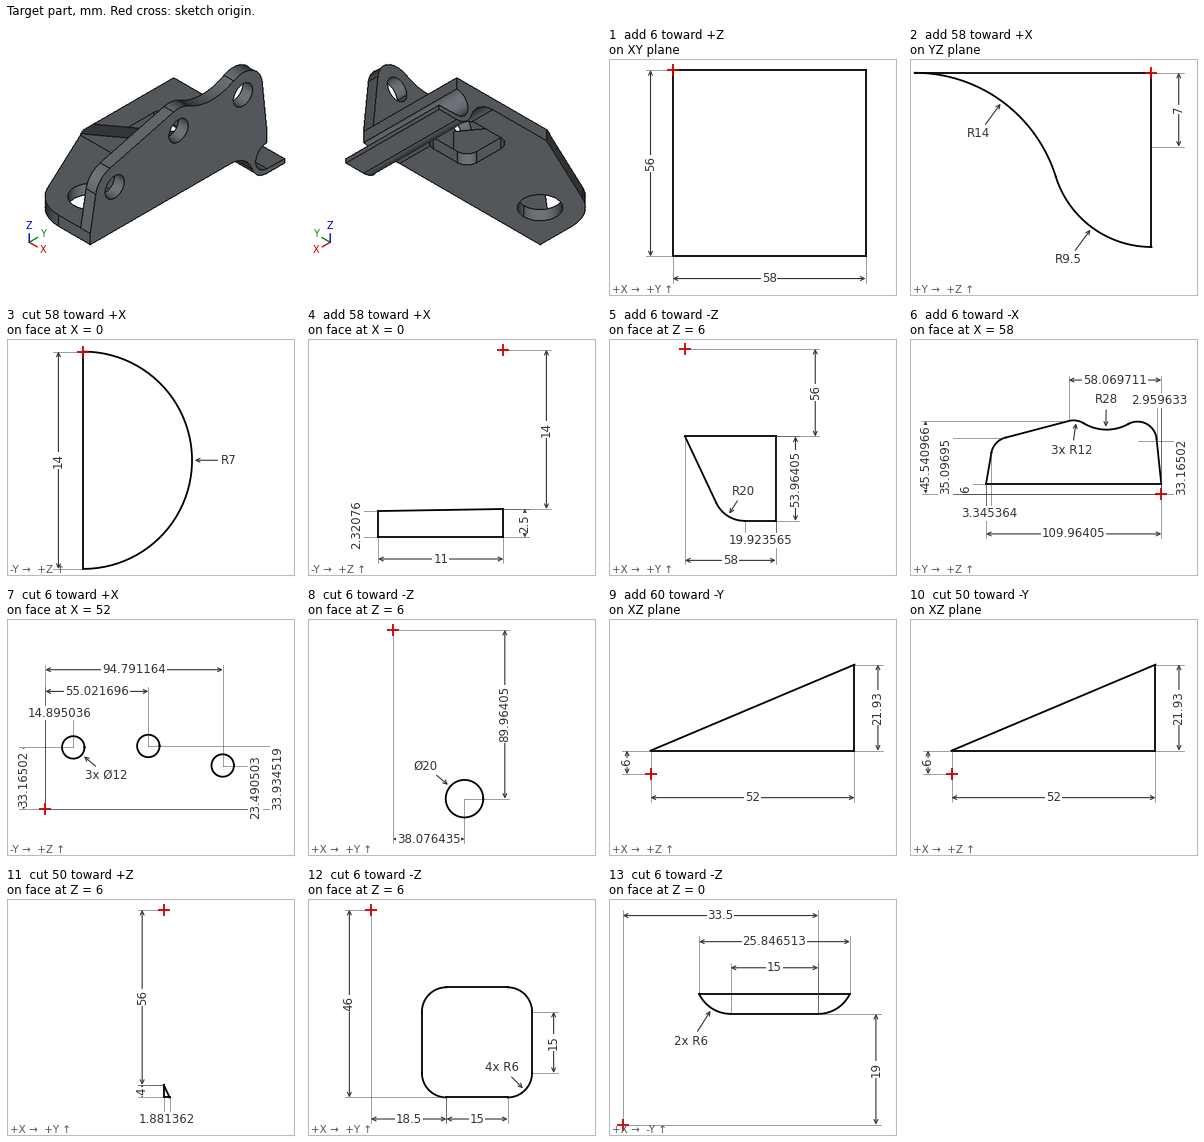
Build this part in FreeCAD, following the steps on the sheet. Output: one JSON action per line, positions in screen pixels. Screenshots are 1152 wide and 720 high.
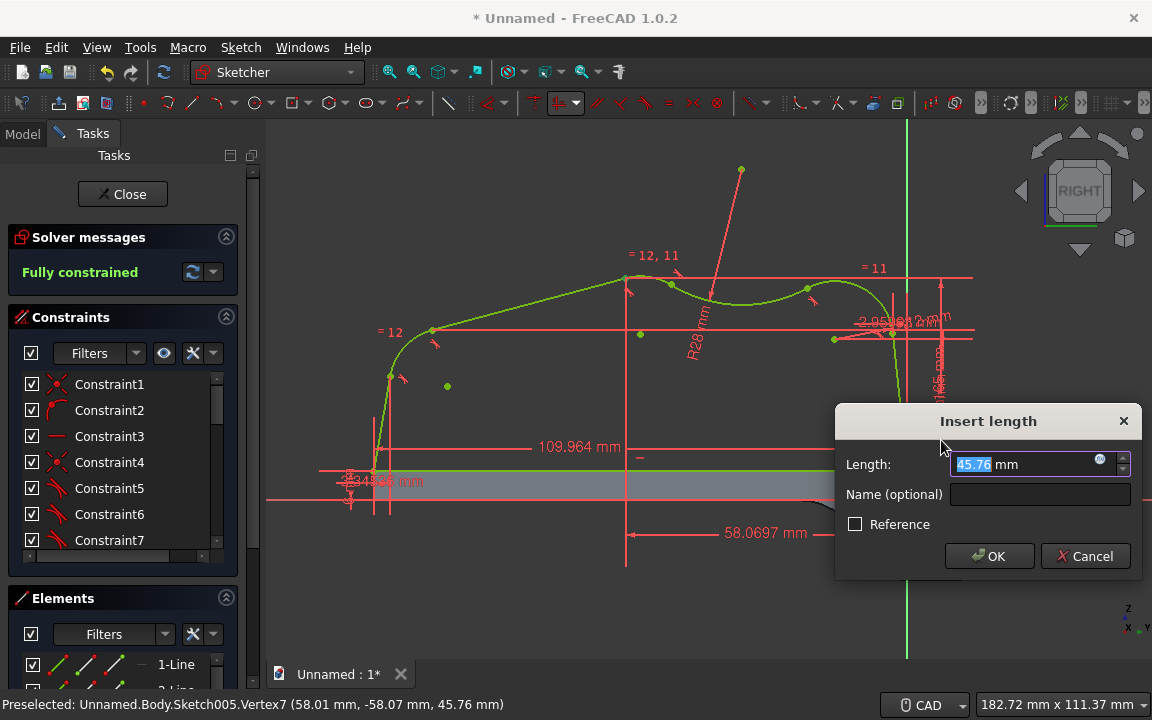
{"action": "type", "text": "45.540966"}
{"action": "key", "text": "Return"}
{"action": "key", "text": "Escape"}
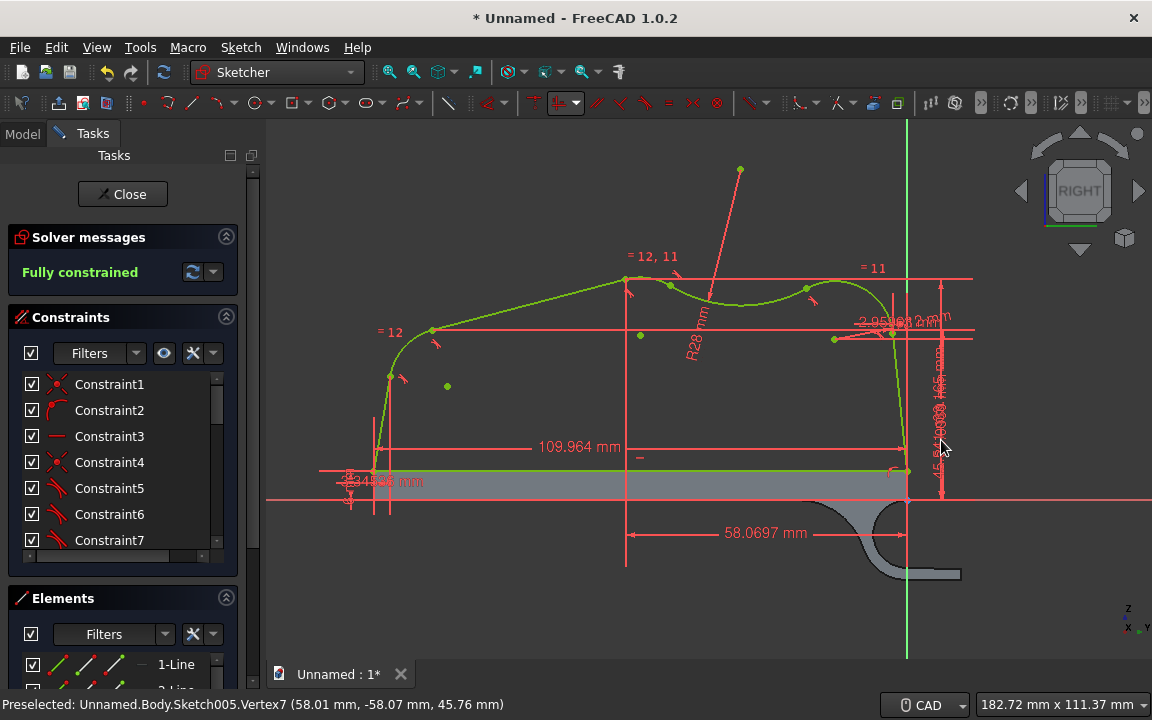
{"action": "left_click", "coordinate": [123, 194]}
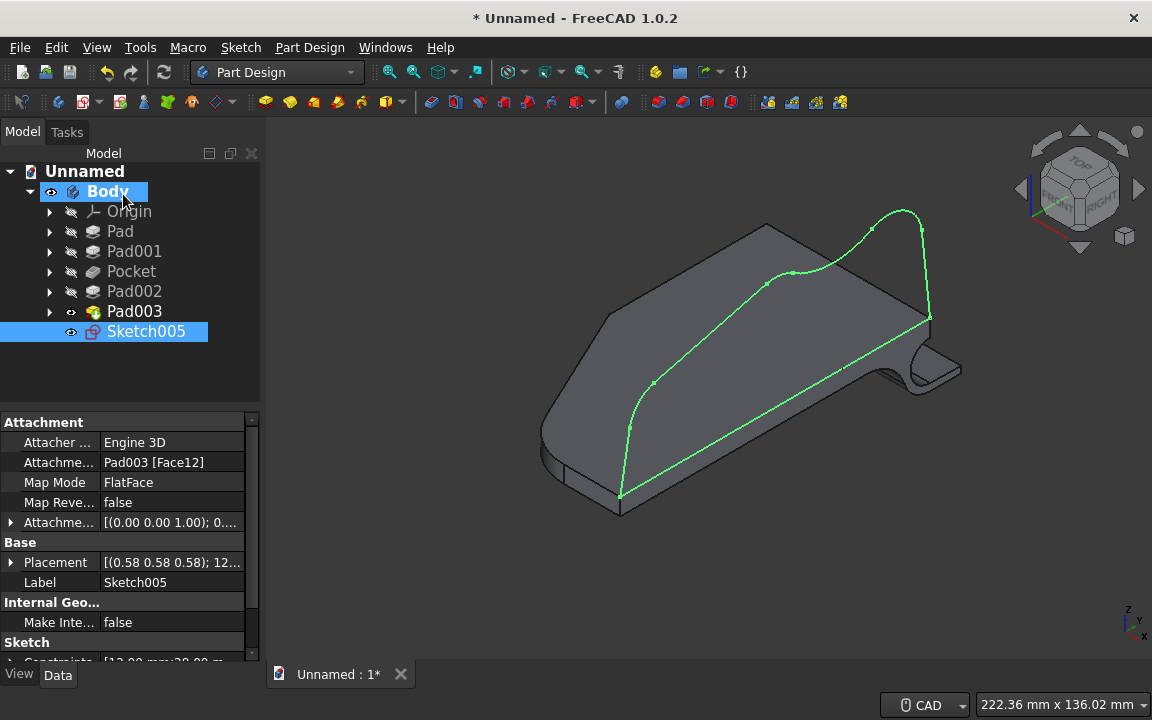
{"action": "left_click", "coordinate": [266, 102]}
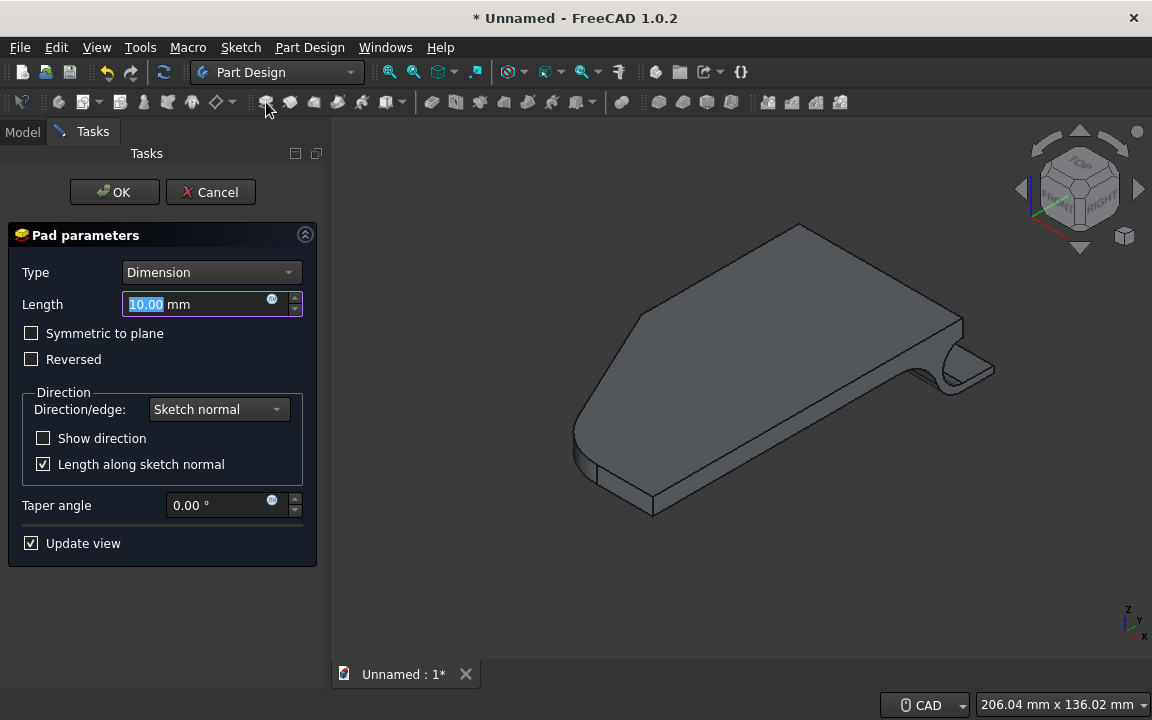
{"action": "type", "text": "6"}
{"action": "key", "text": "Tab"}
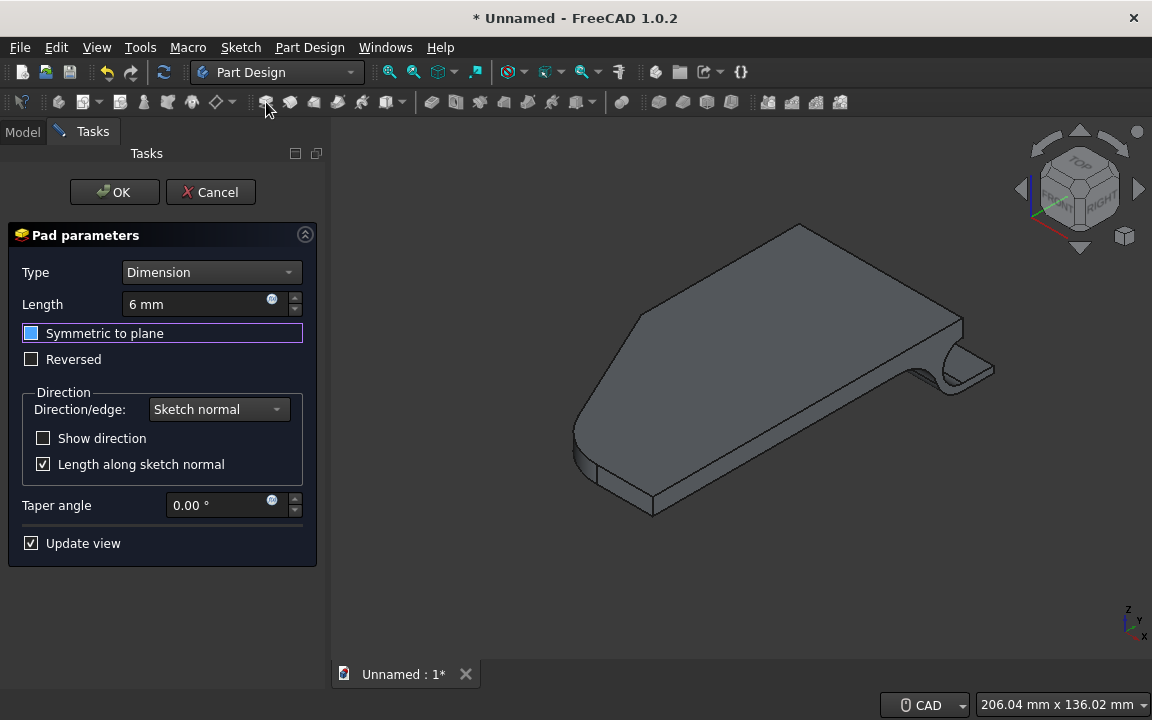
{"action": "left_click", "coordinate": [30, 359]}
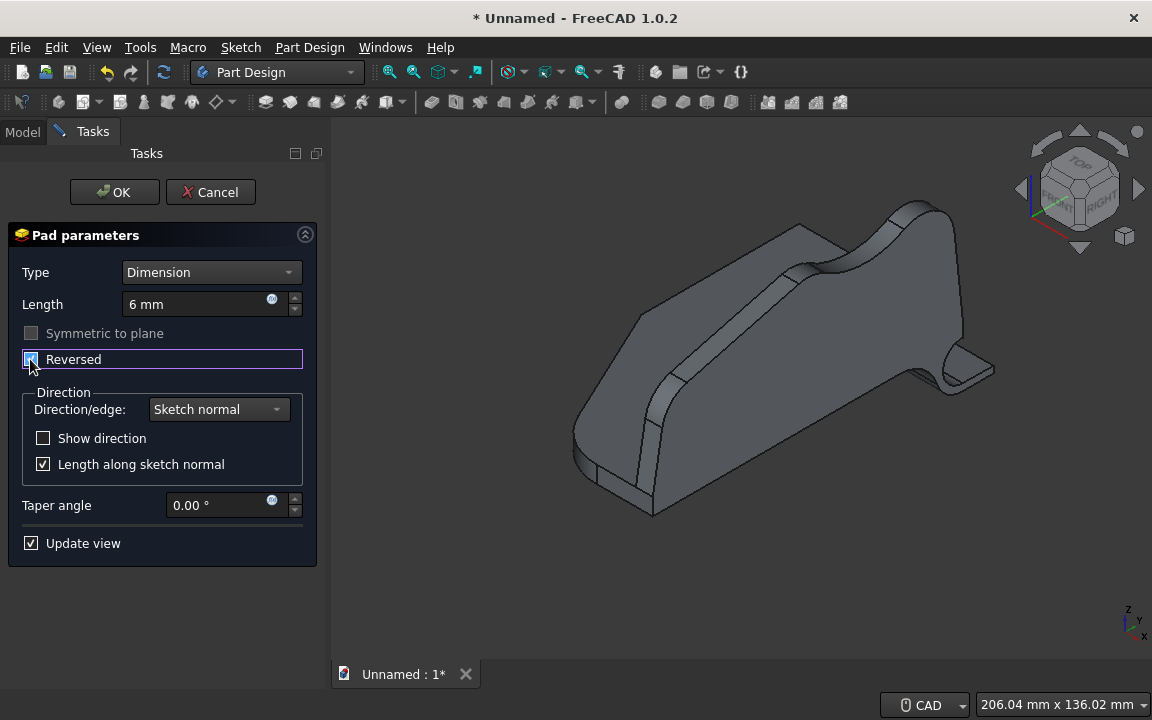
{"action": "left_click", "coordinate": [115, 192]}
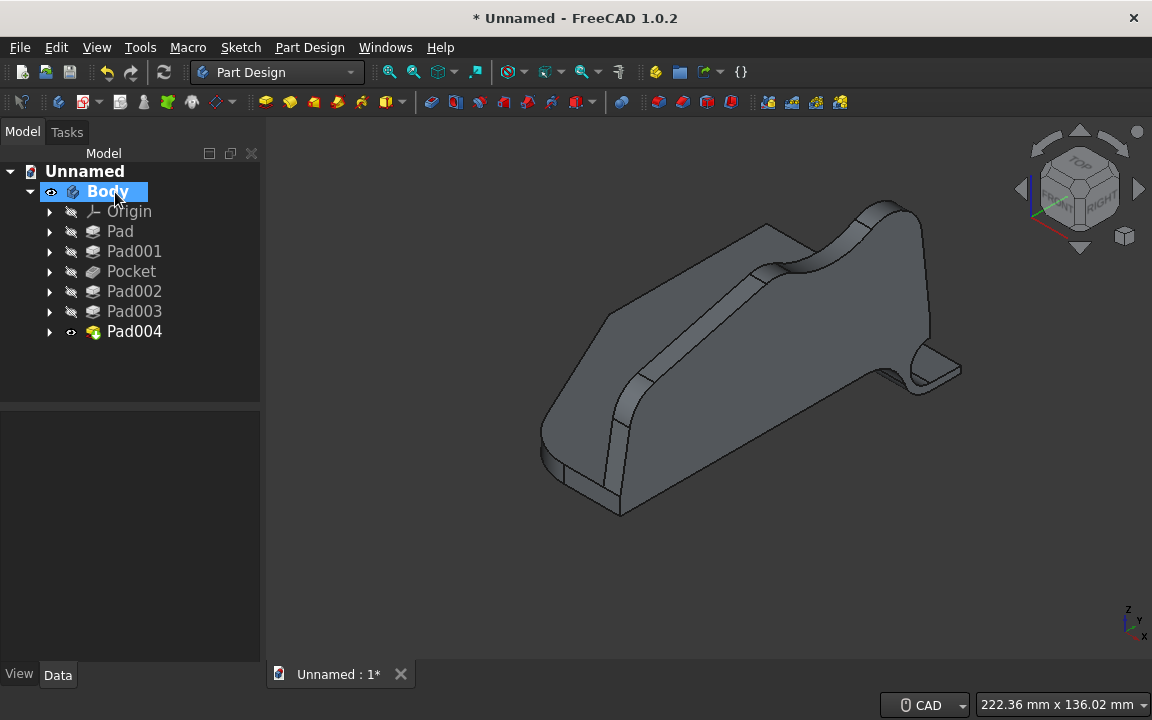
{"action": "left_click", "coordinate": [390, 72]}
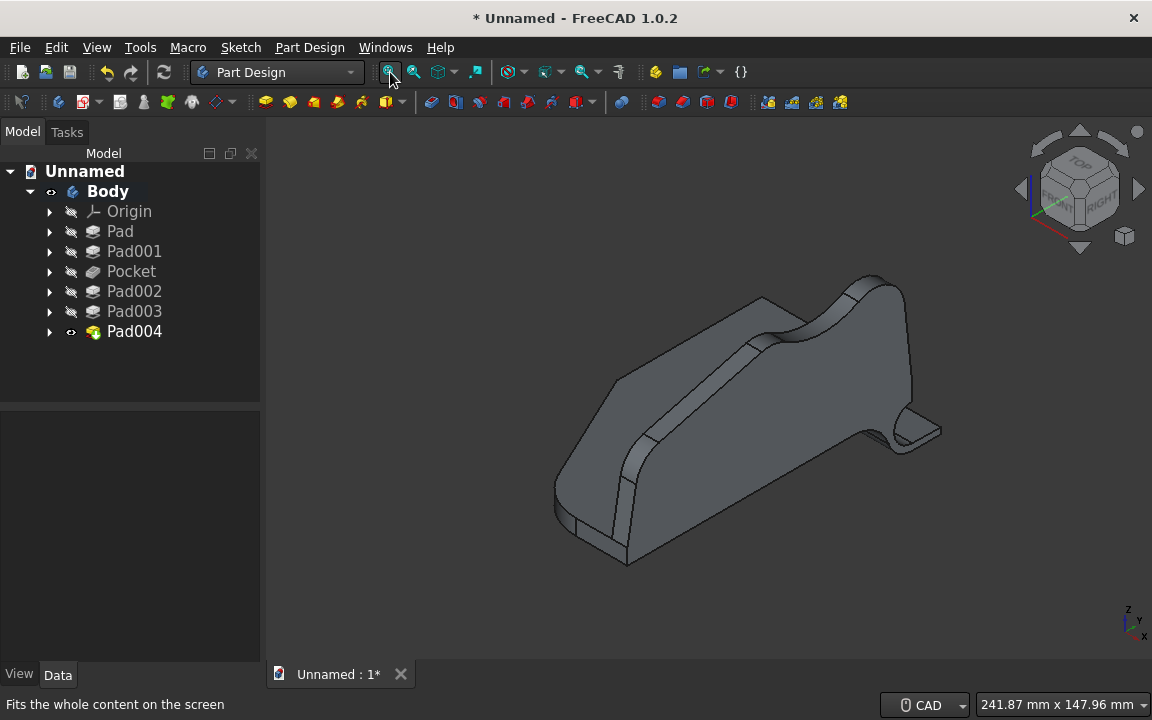
{"action": "key", "text": "6"}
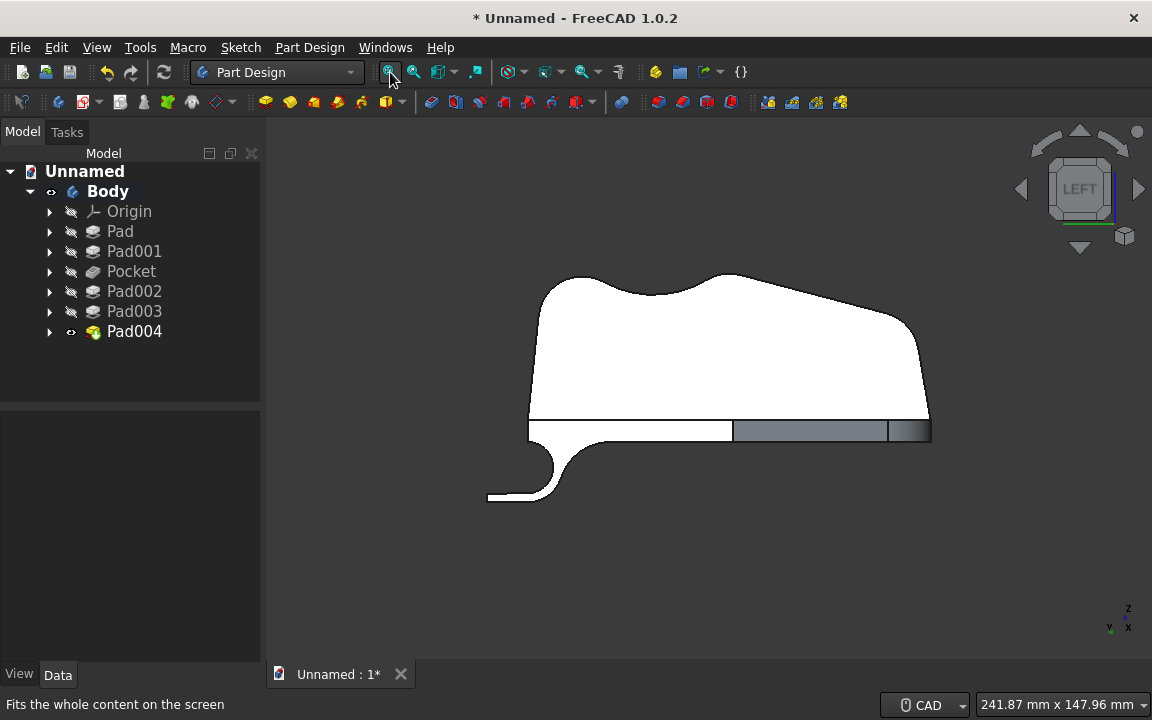
{"action": "left_click", "coordinate": [729, 346]}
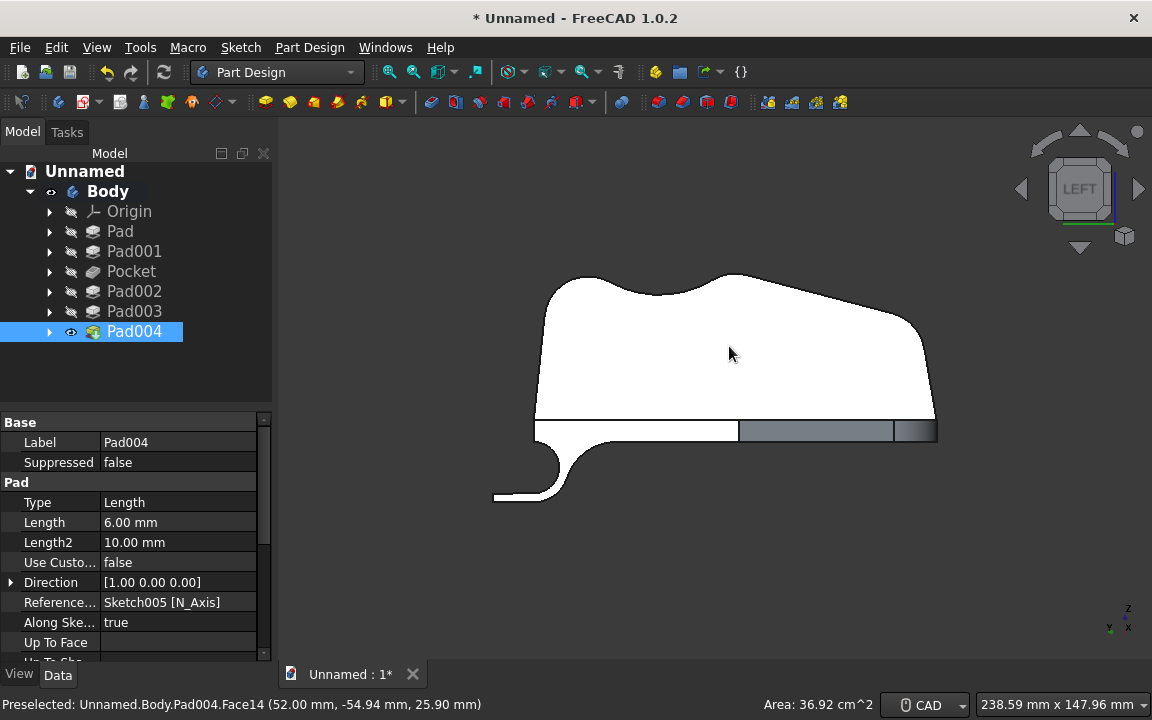
{"action": "left_click", "coordinate": [84, 102]}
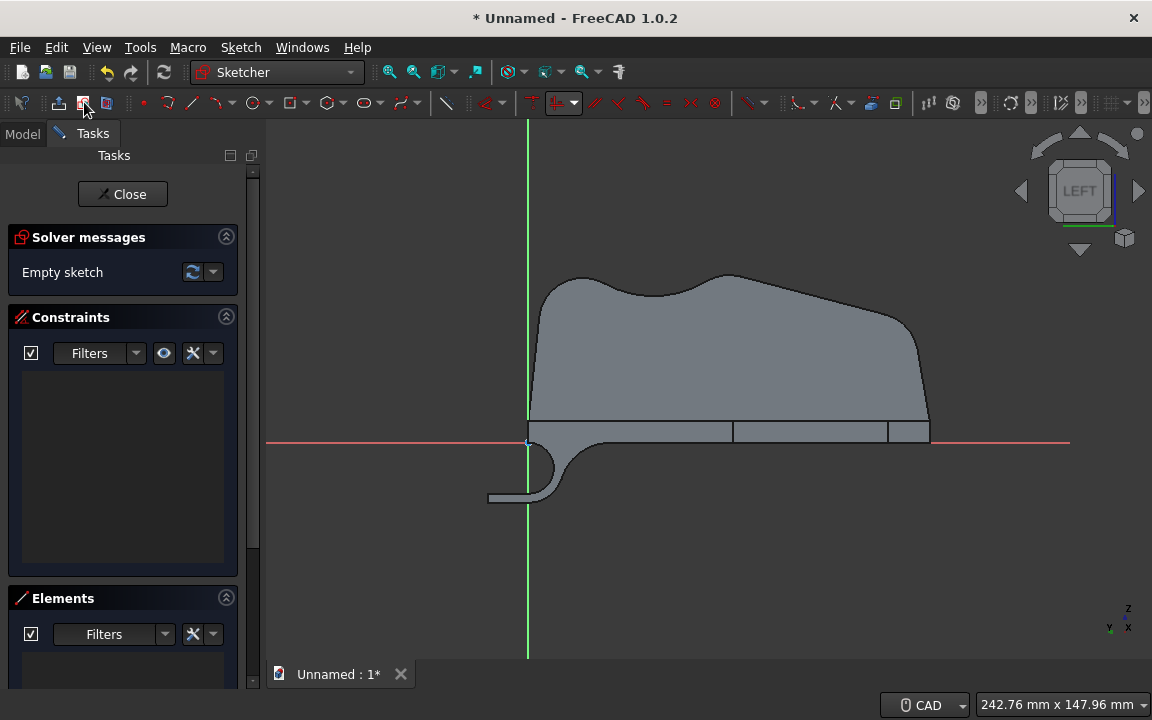
{"action": "key", "text": "q s"}